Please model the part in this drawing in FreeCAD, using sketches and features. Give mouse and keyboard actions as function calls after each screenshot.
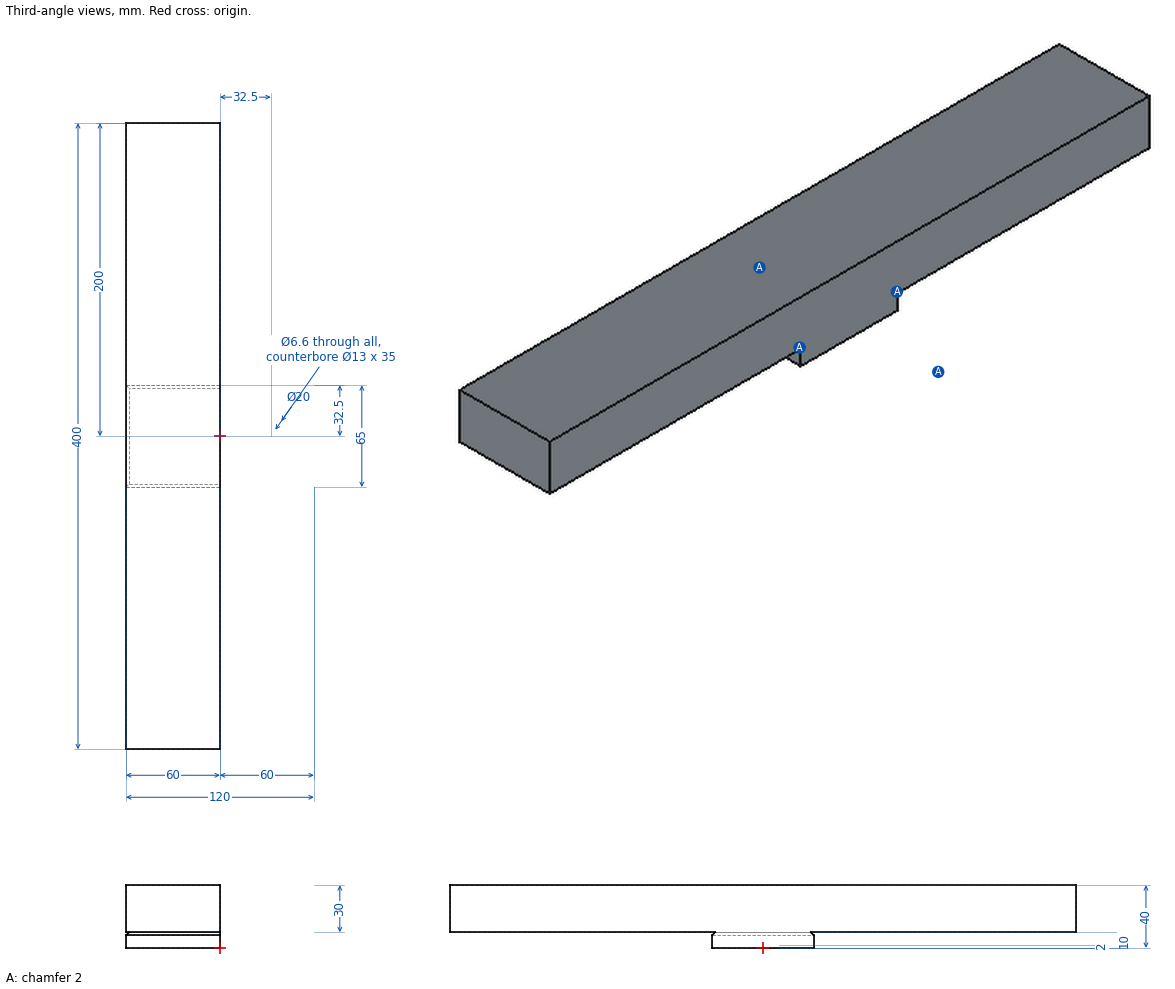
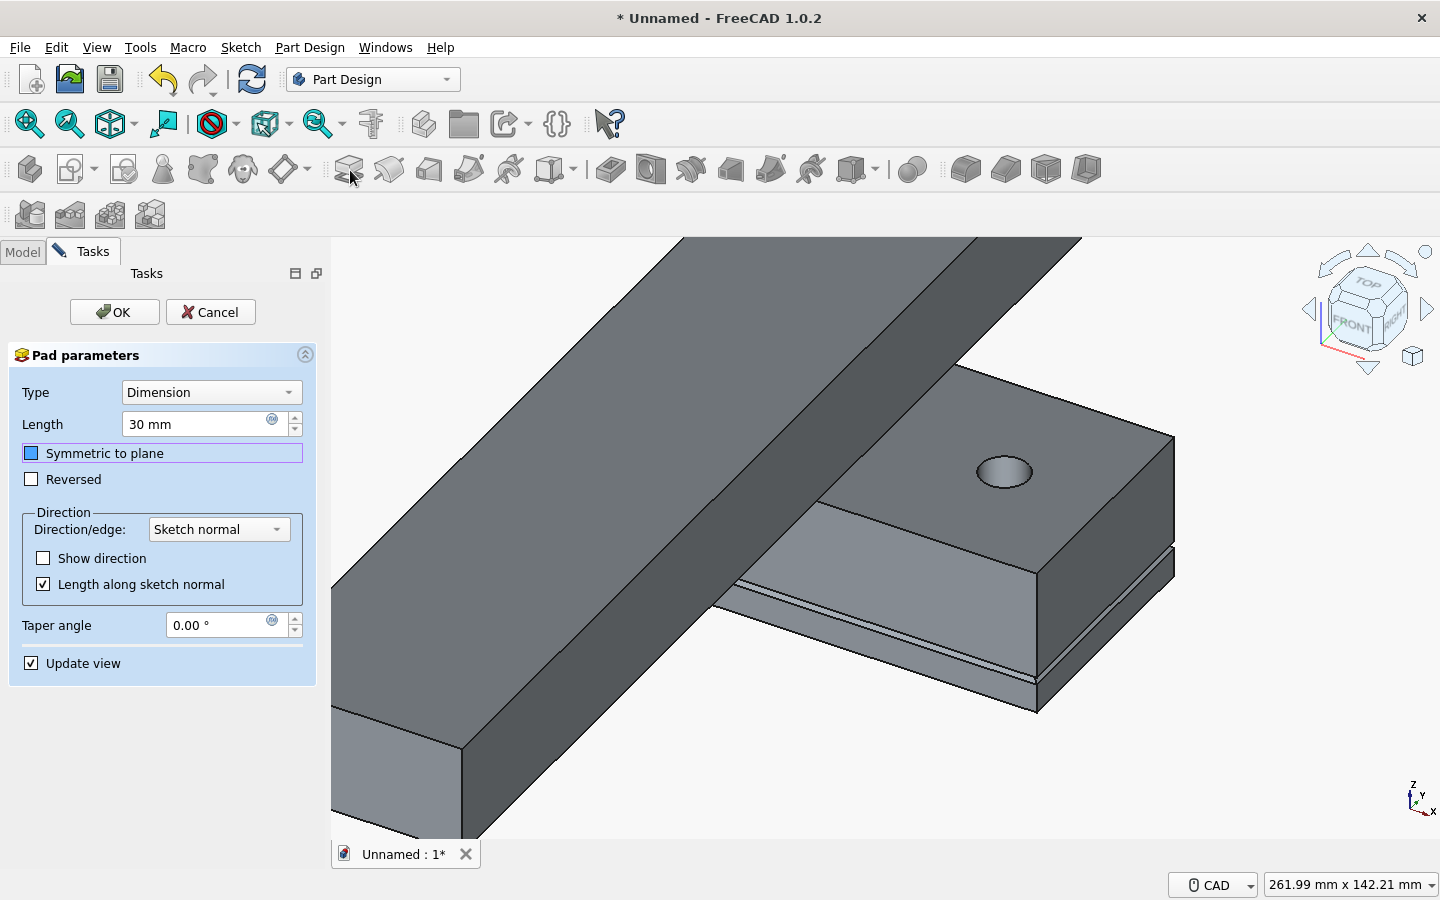
click(30, 479)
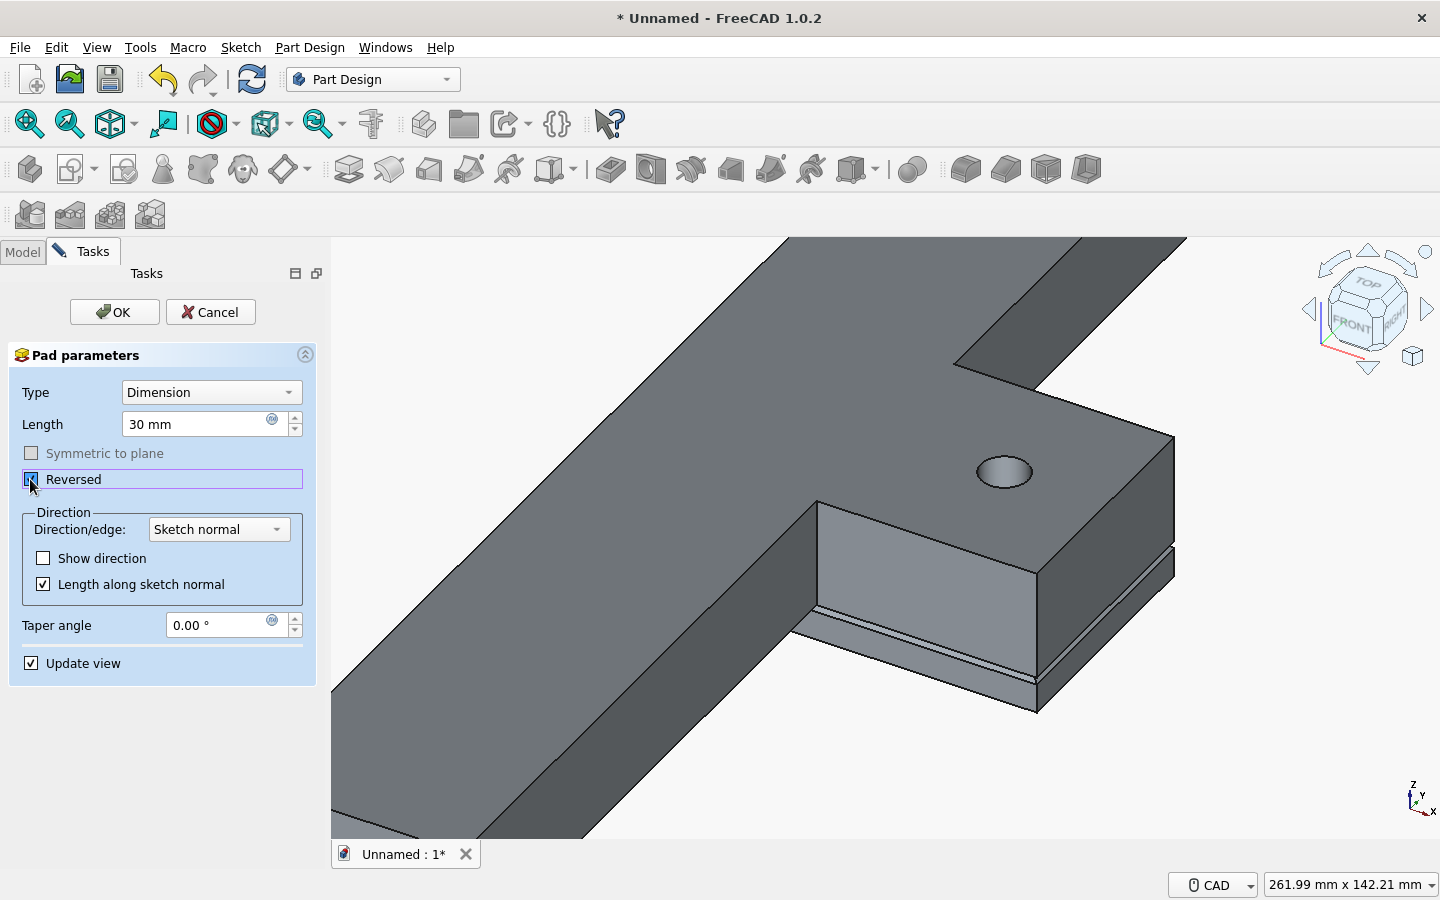
click(115, 312)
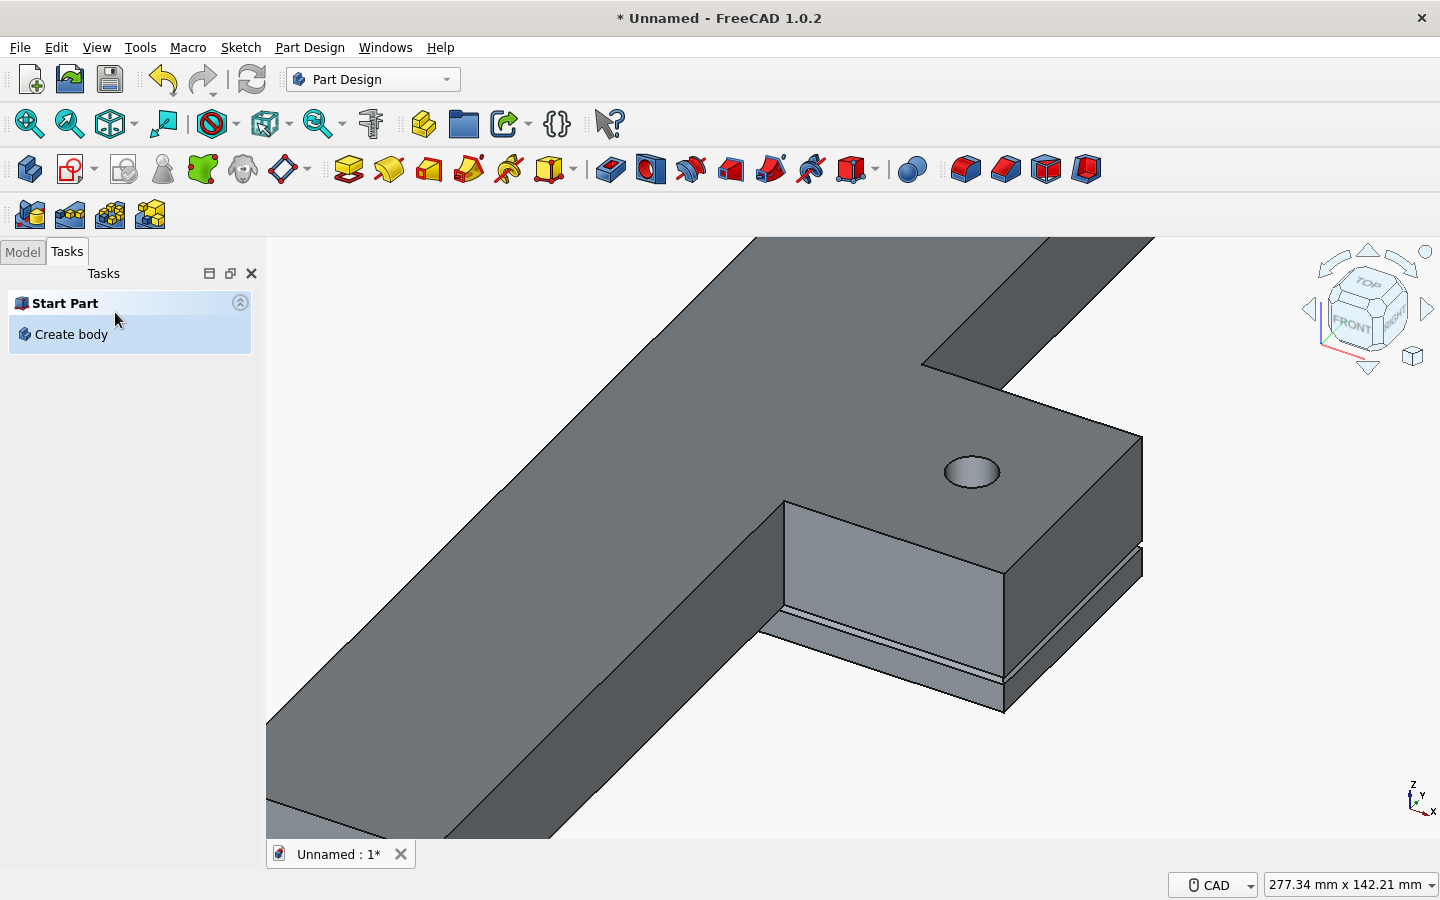
click(30, 124)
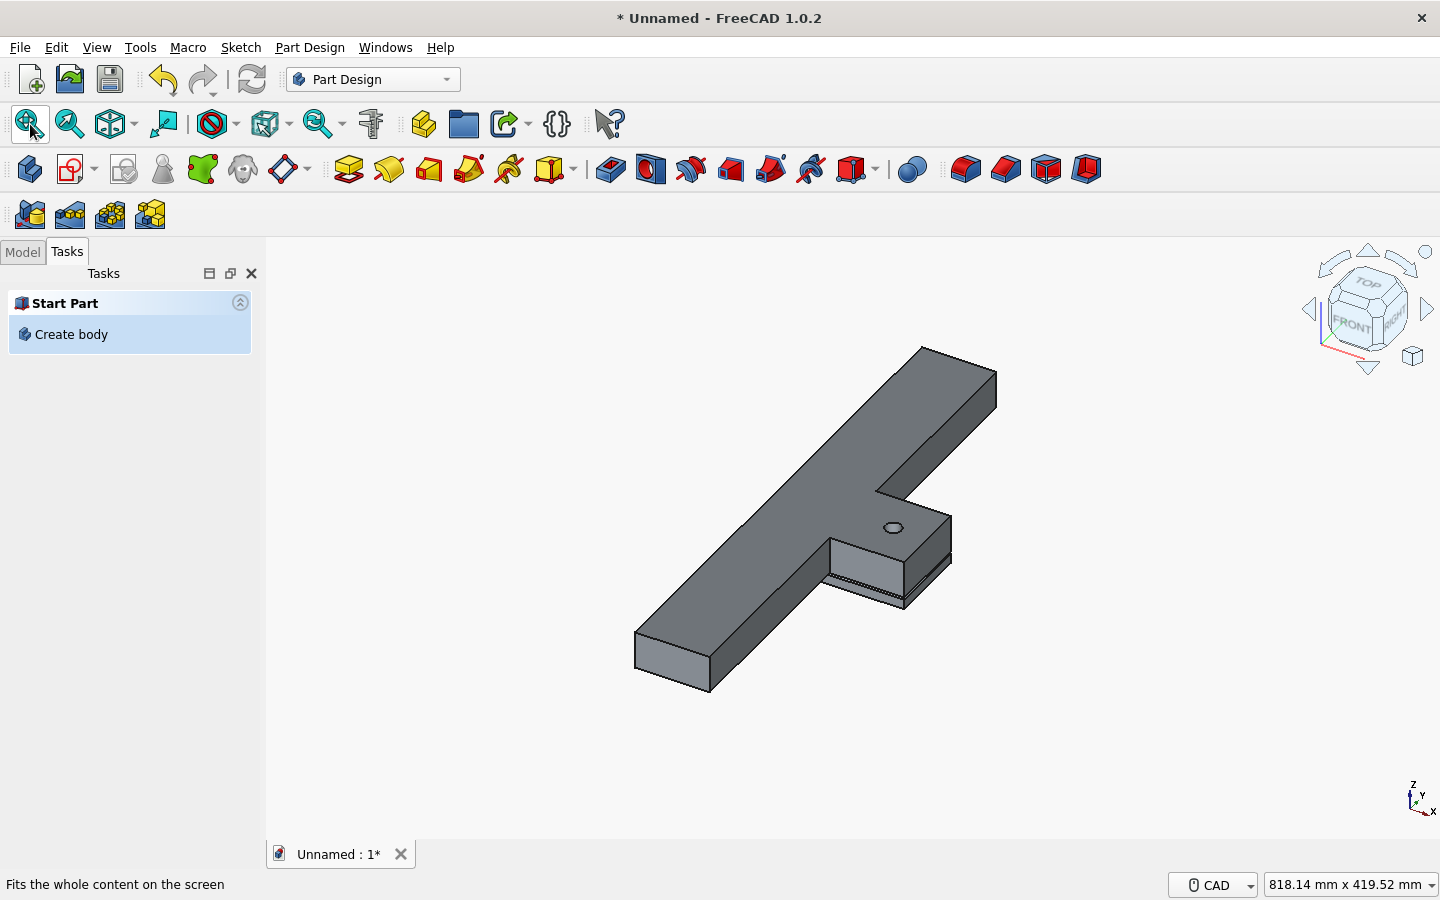
click(832, 506)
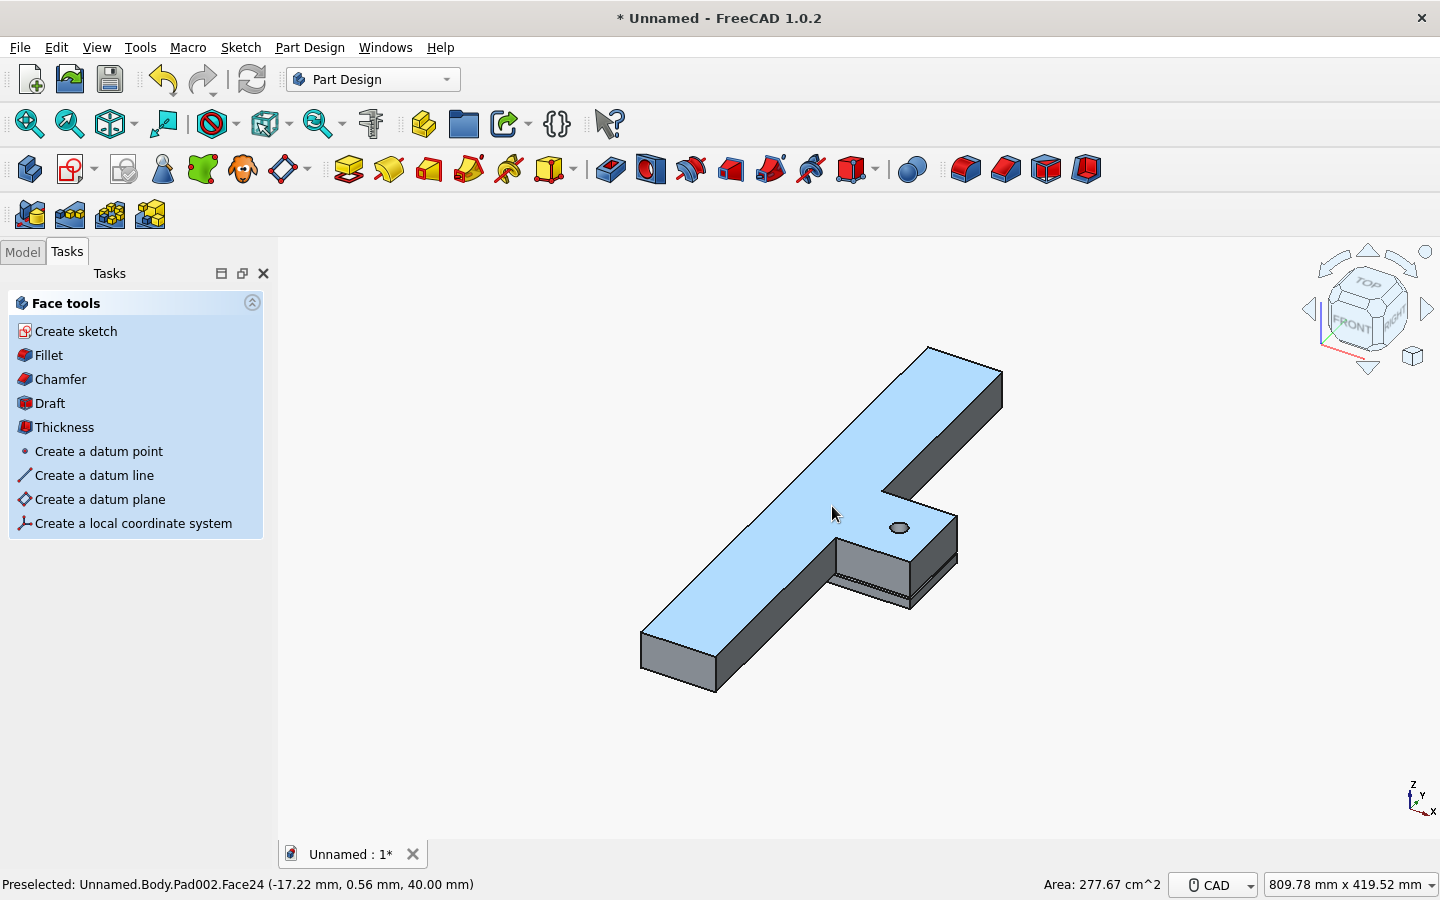
click(70, 170)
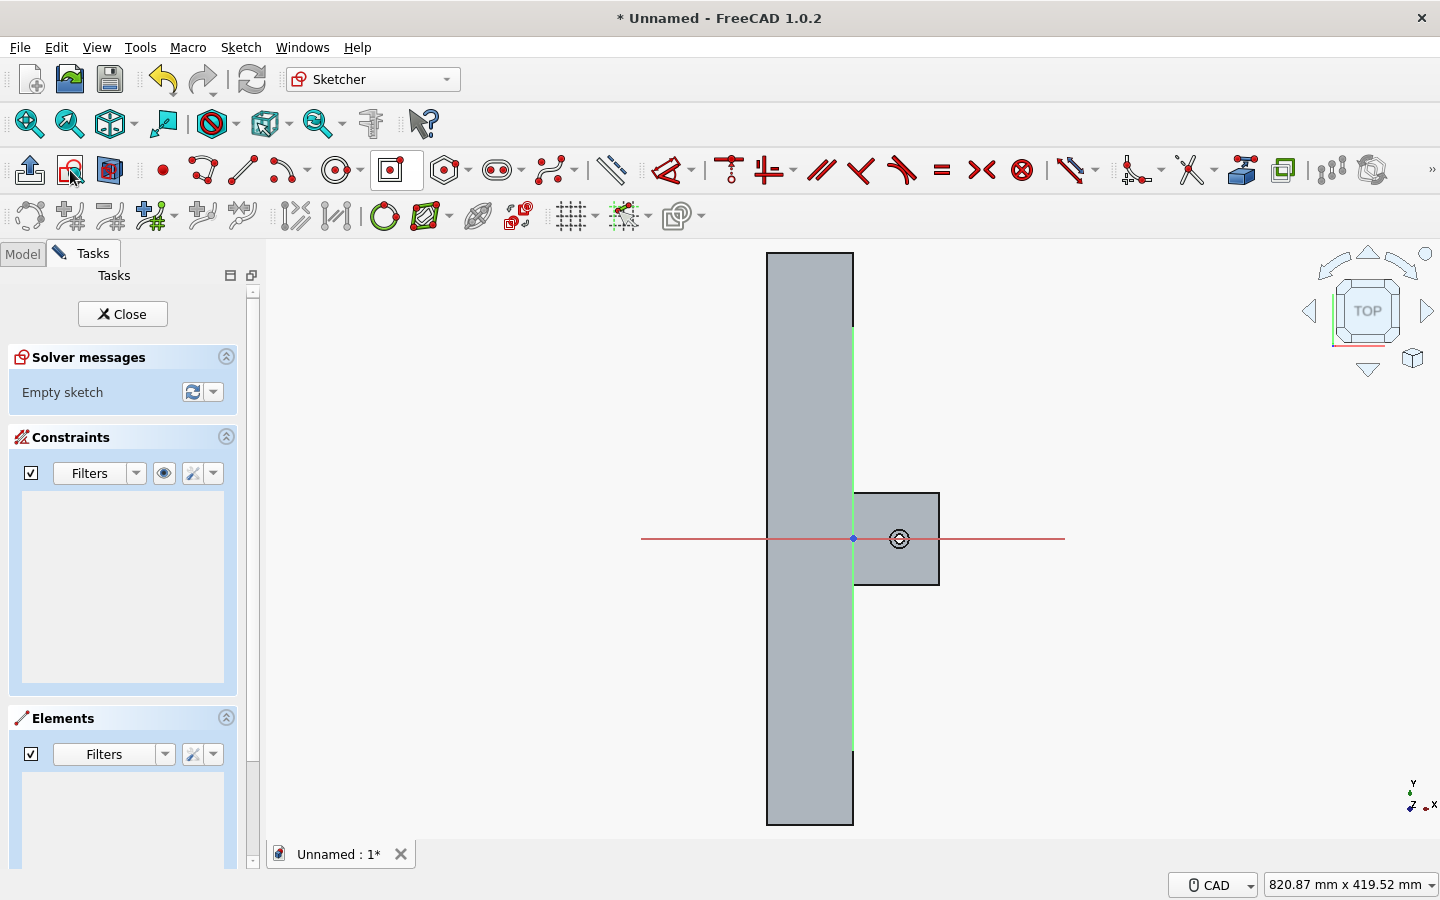
scroll(932, 539, up, 7)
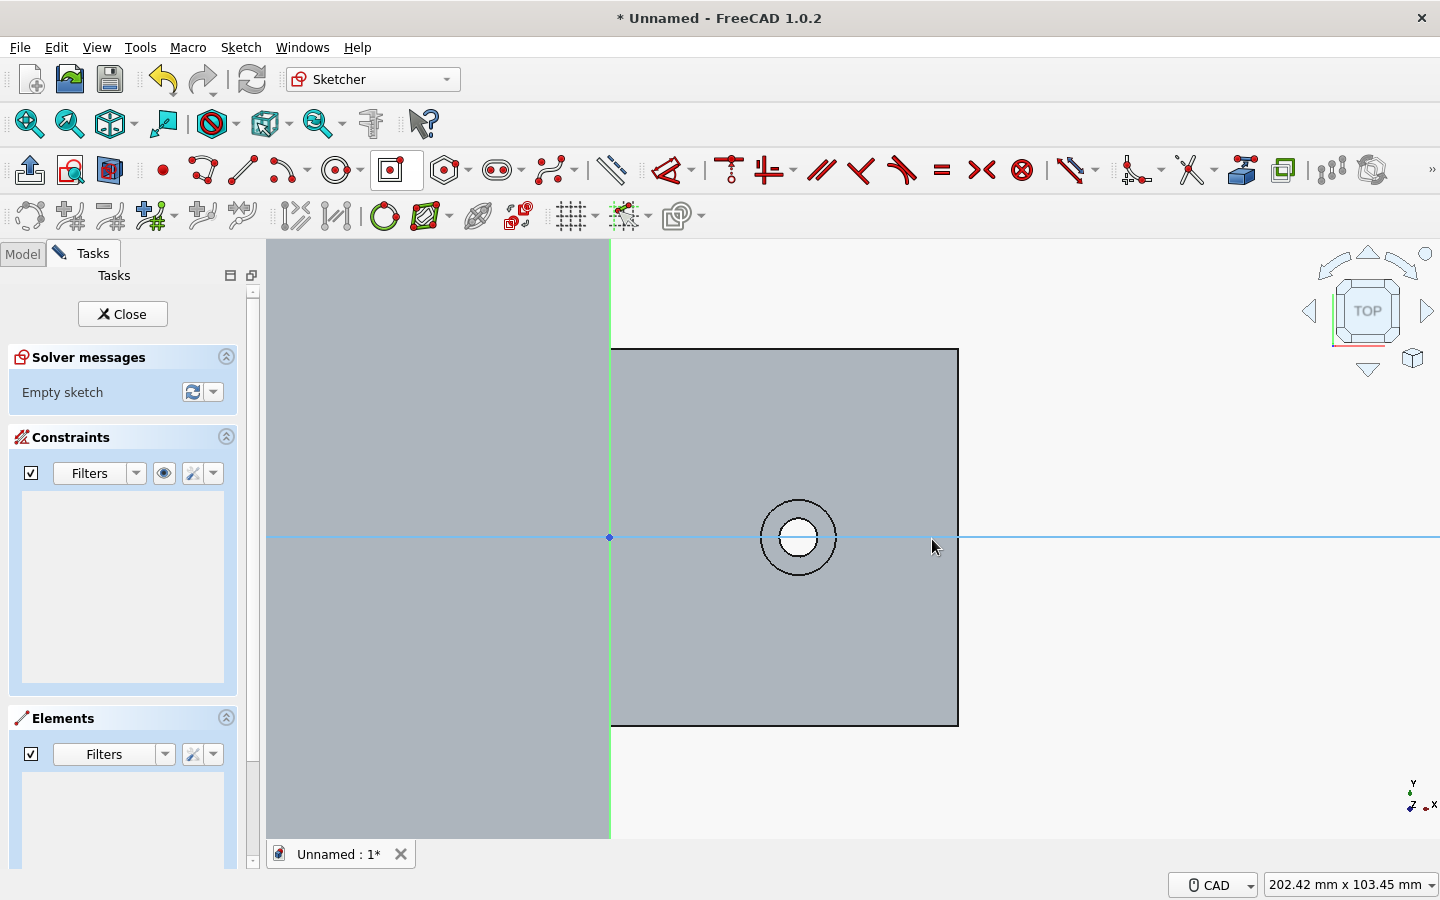
key(g)
key(r)